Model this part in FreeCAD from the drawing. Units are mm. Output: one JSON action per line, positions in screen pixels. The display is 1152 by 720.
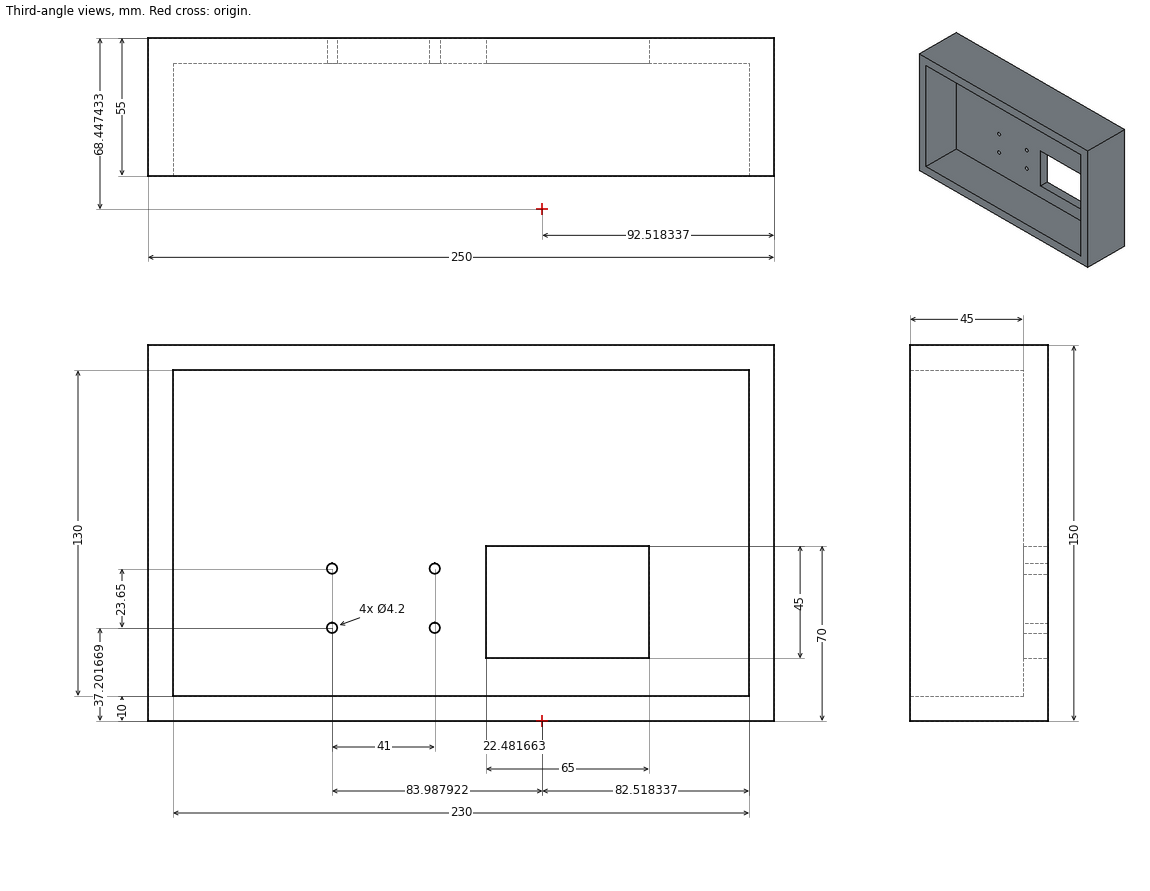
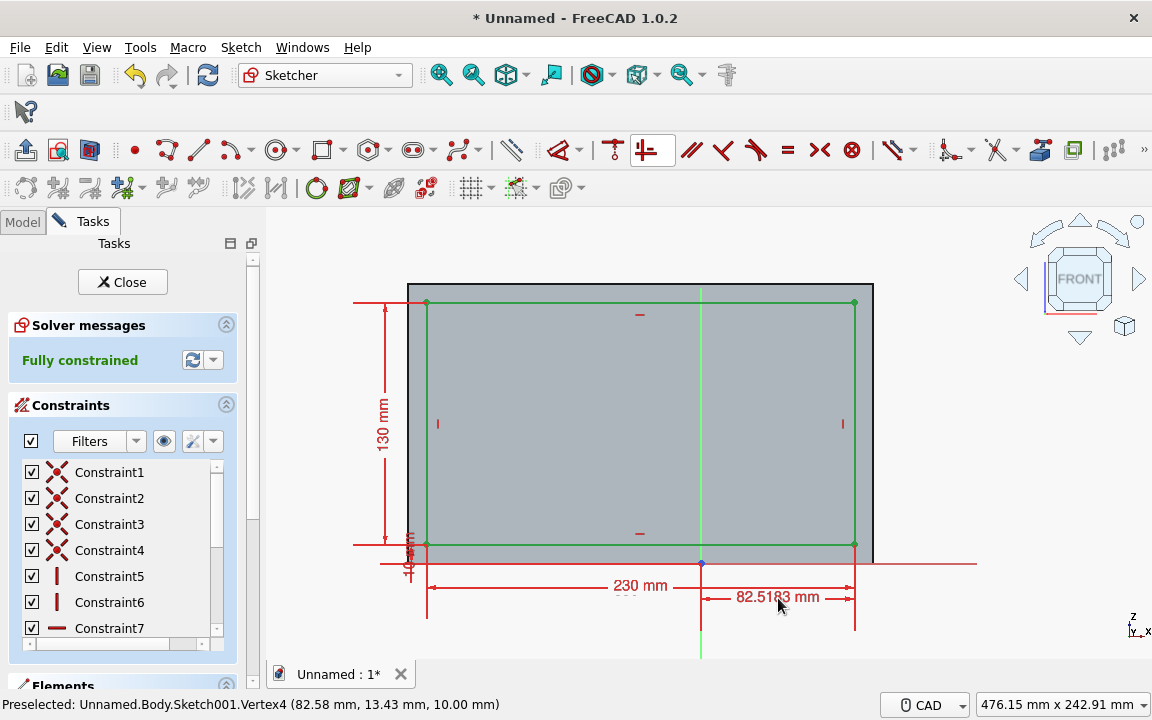
{"action": "left_click", "coordinate": [123, 282]}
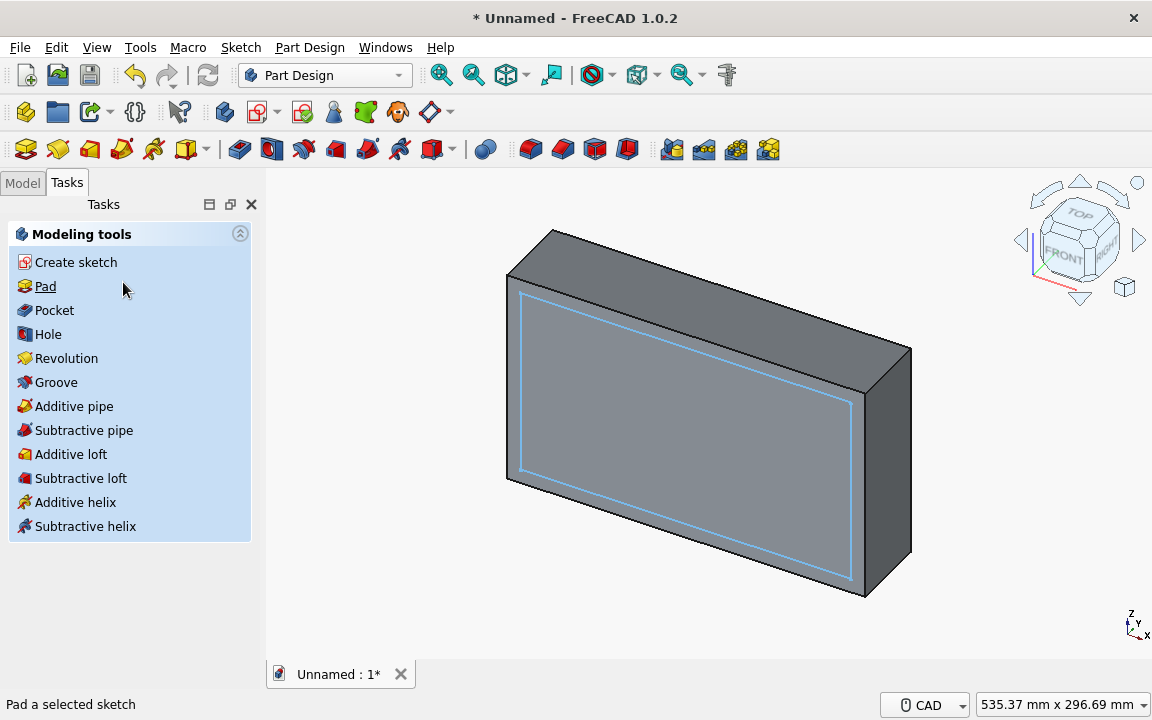
{"action": "left_click", "coordinate": [240, 150]}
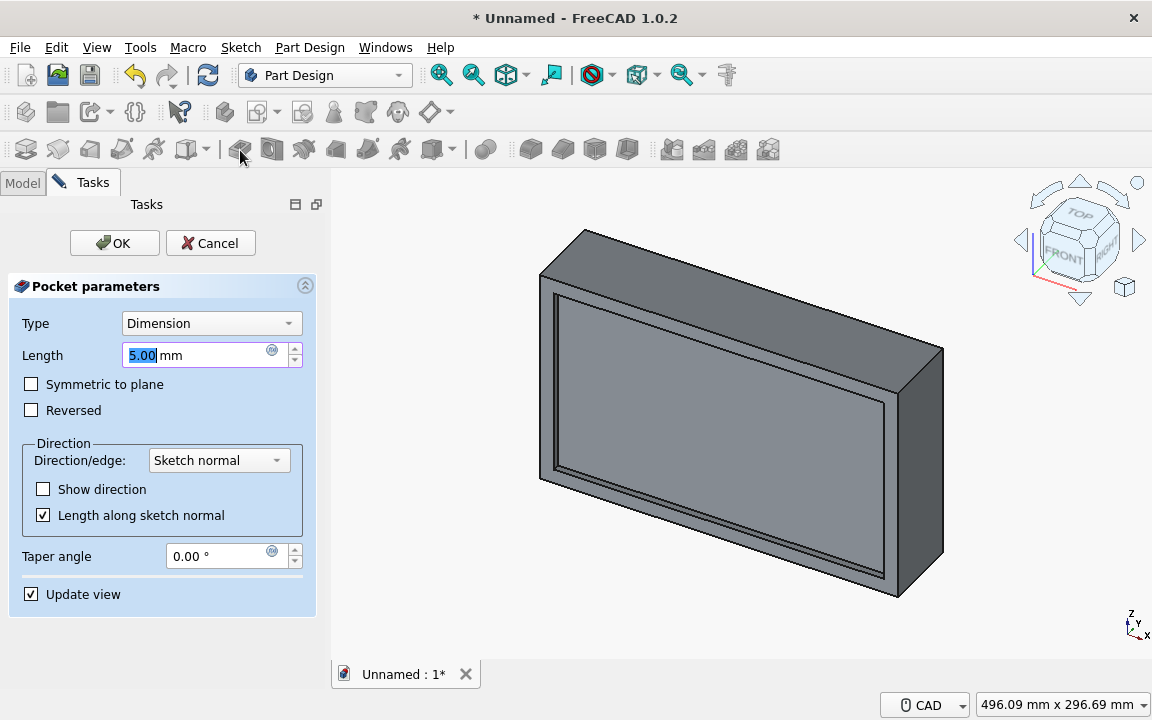
{"action": "type", "text": "45"}
{"action": "key", "text": "Tab"}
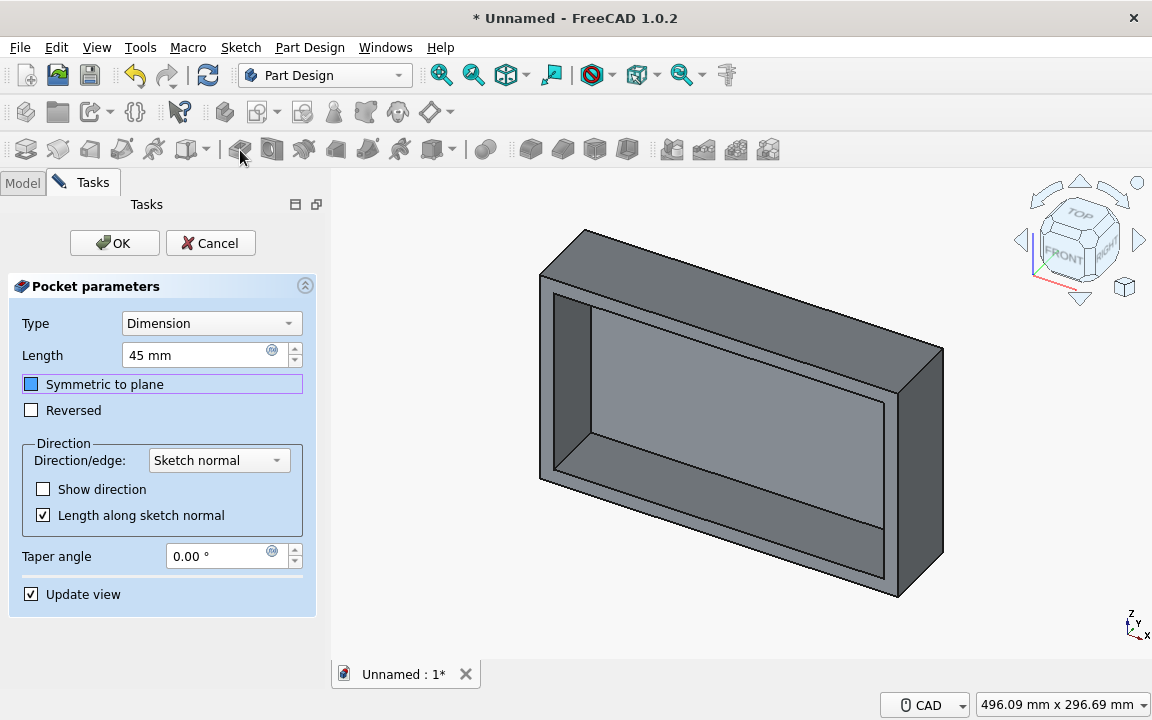
{"action": "left_click", "coordinate": [115, 243]}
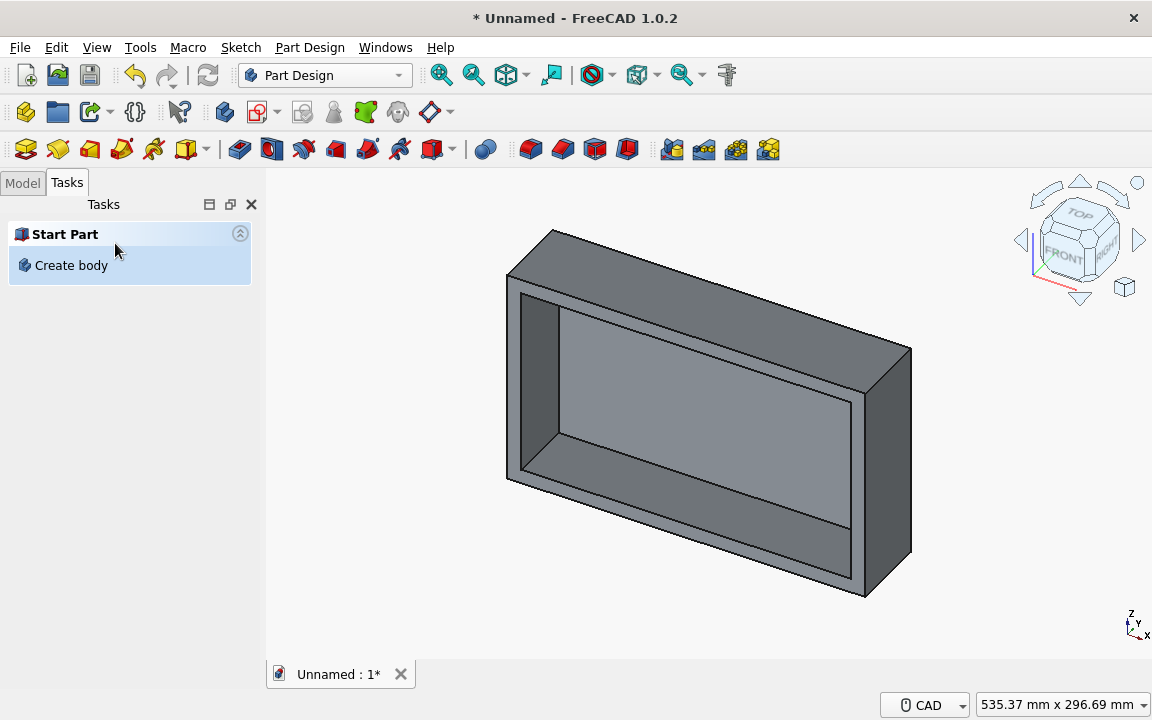
{"action": "left_click", "coordinate": [771, 414]}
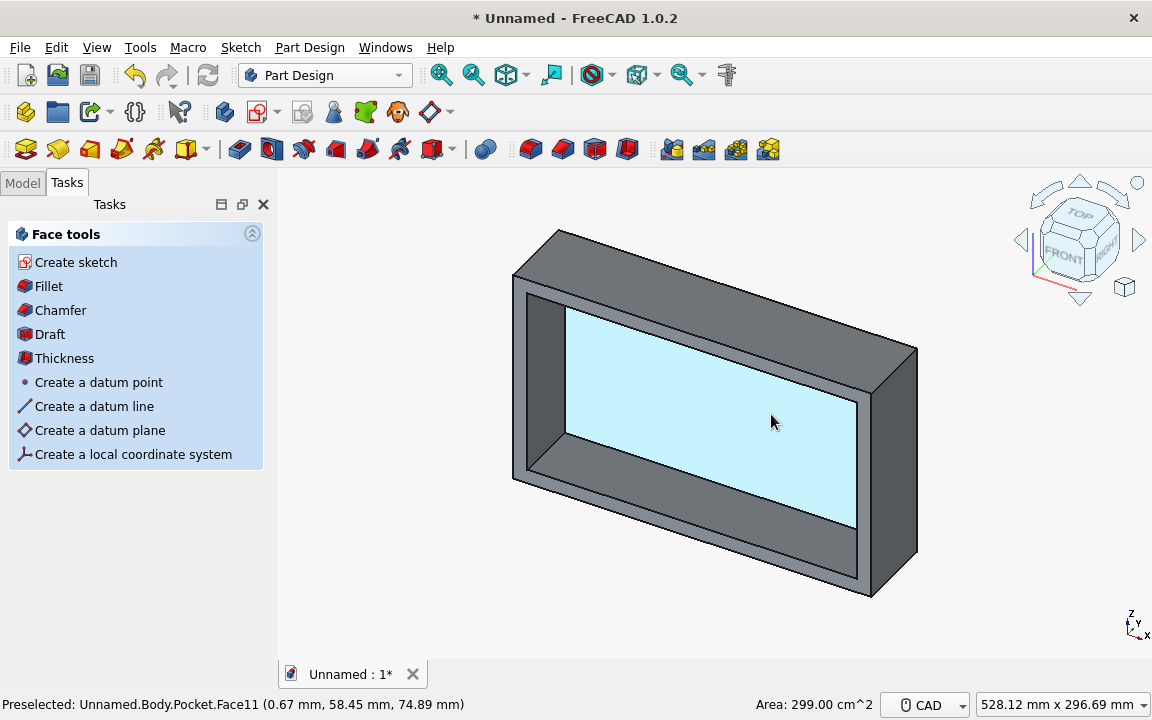
{"action": "left_click", "coordinate": [258, 112]}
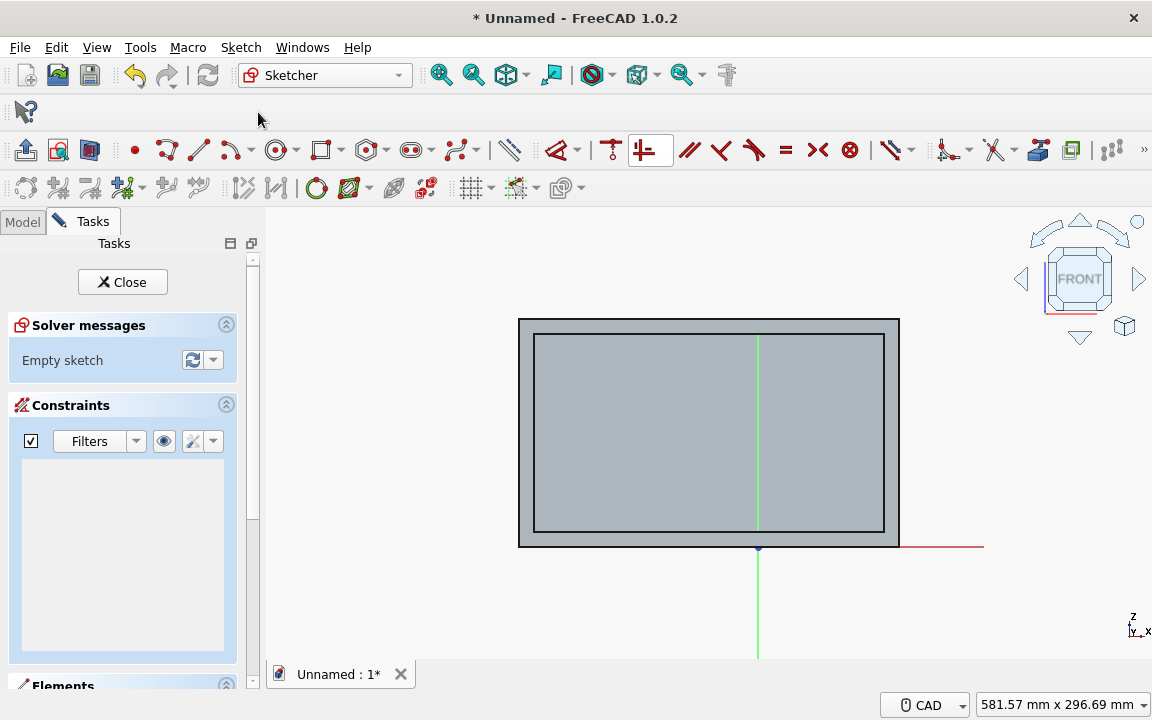
{"action": "scroll", "coordinate": [851, 529], "scroll_direction": "up", "scroll_amount": 5}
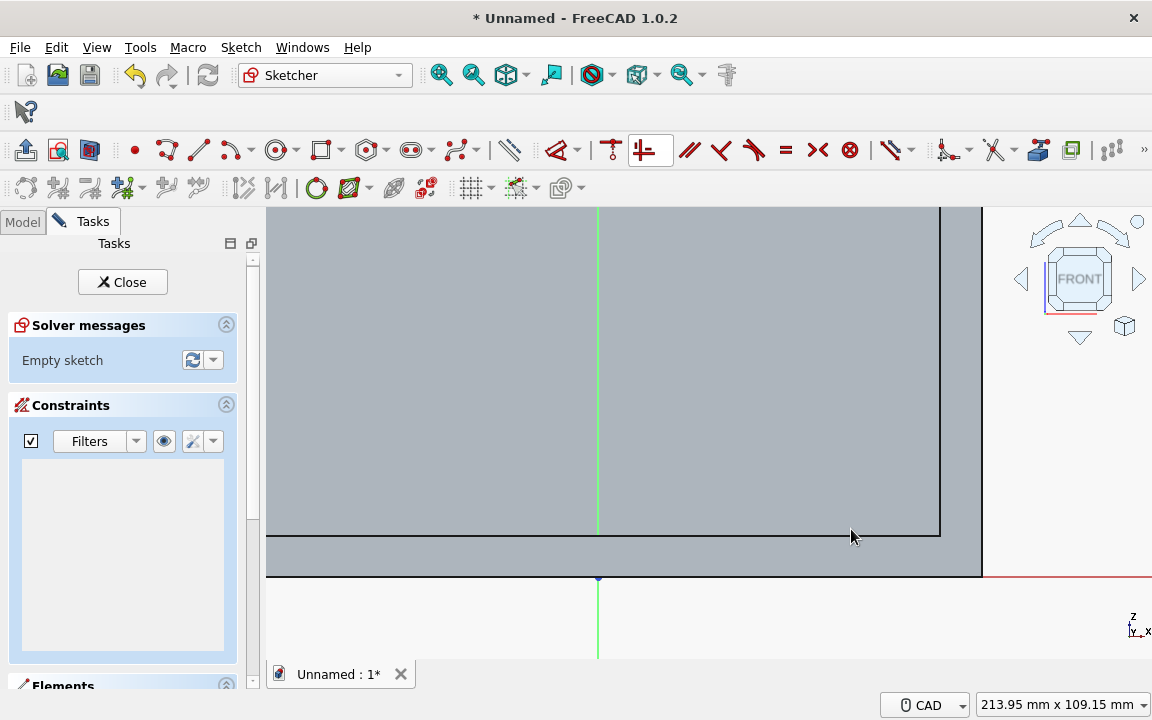
{"action": "left_click", "coordinate": [322, 150]}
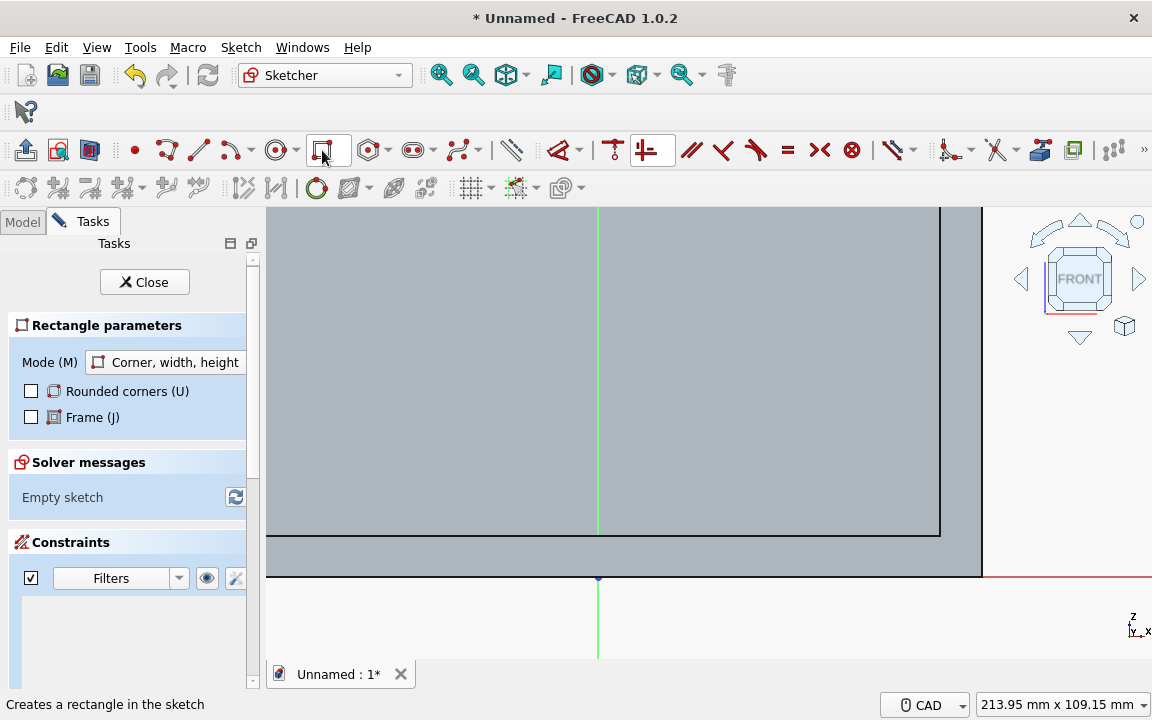
{"action": "left_click", "coordinate": [505, 288]}
{"action": "left_click", "coordinate": [774, 474]}
{"action": "key", "text": "Escape"}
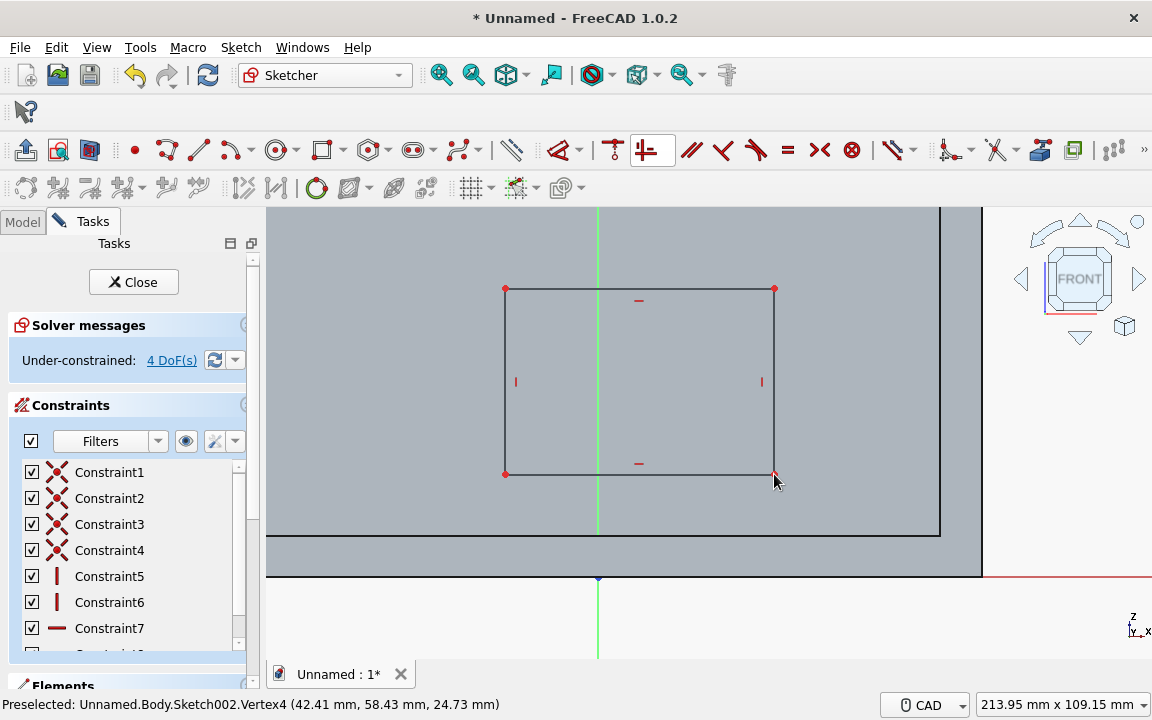
{"action": "left_click", "coordinate": [558, 150]}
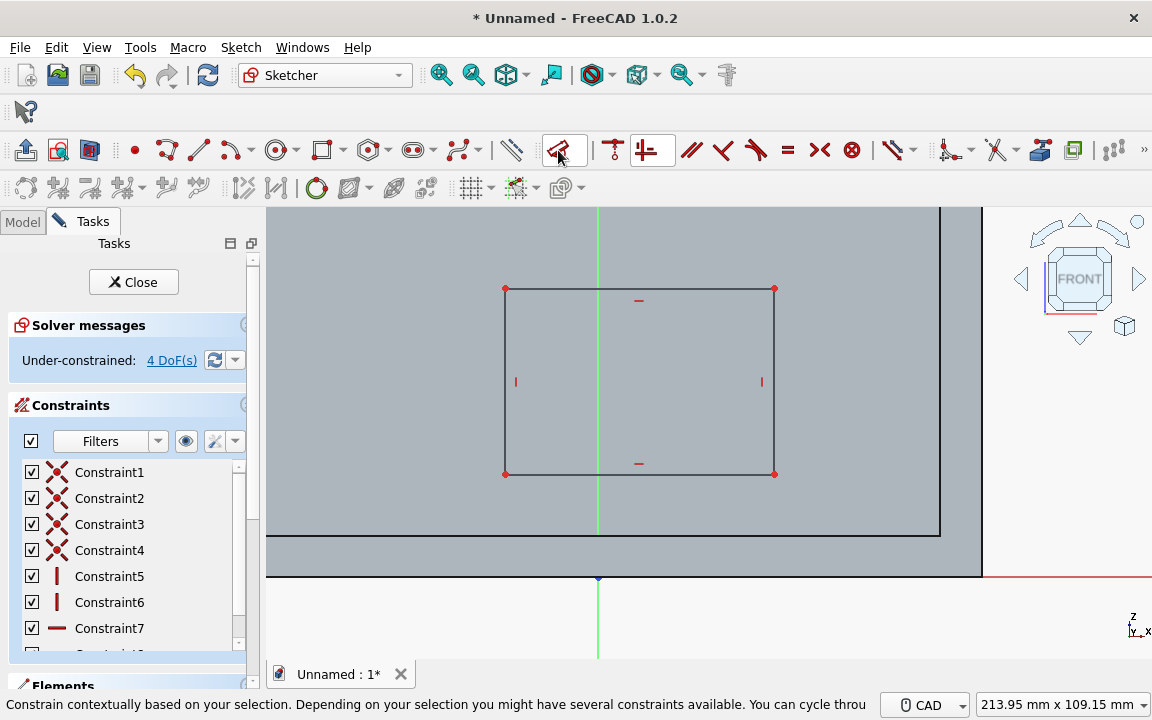
{"action": "left_click", "coordinate": [505, 345]}
{"action": "left_click", "coordinate": [471, 382]}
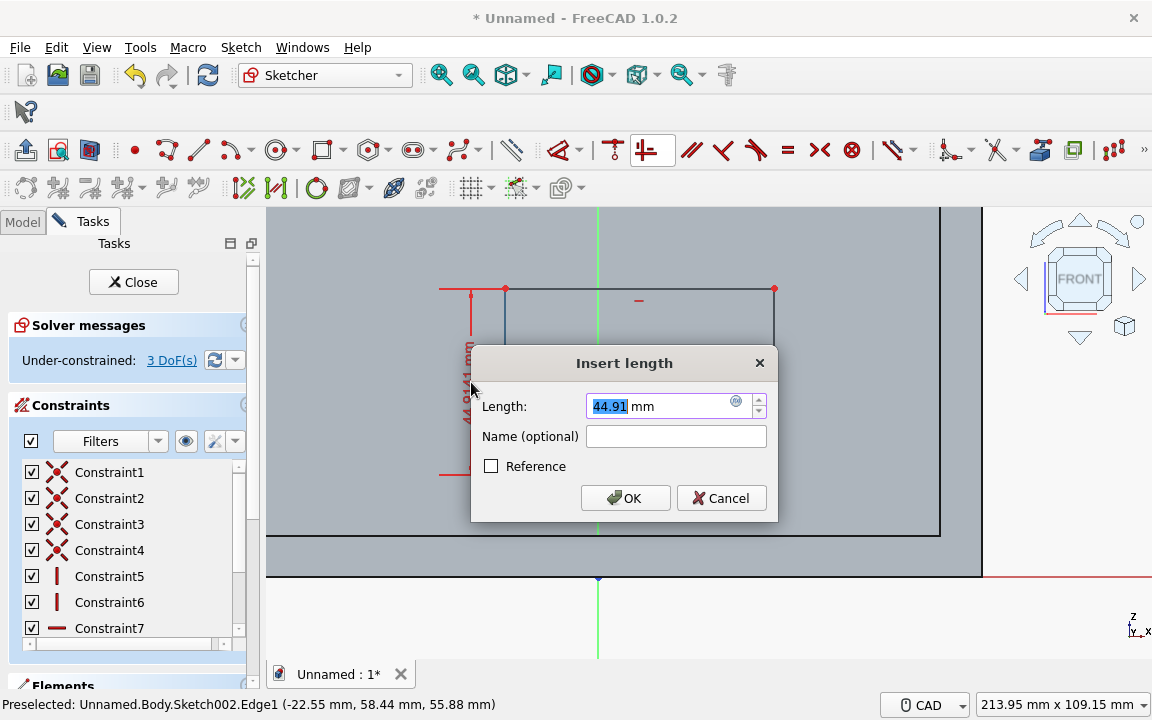
{"action": "type", "text": "45"}
{"action": "key", "text": "Return"}